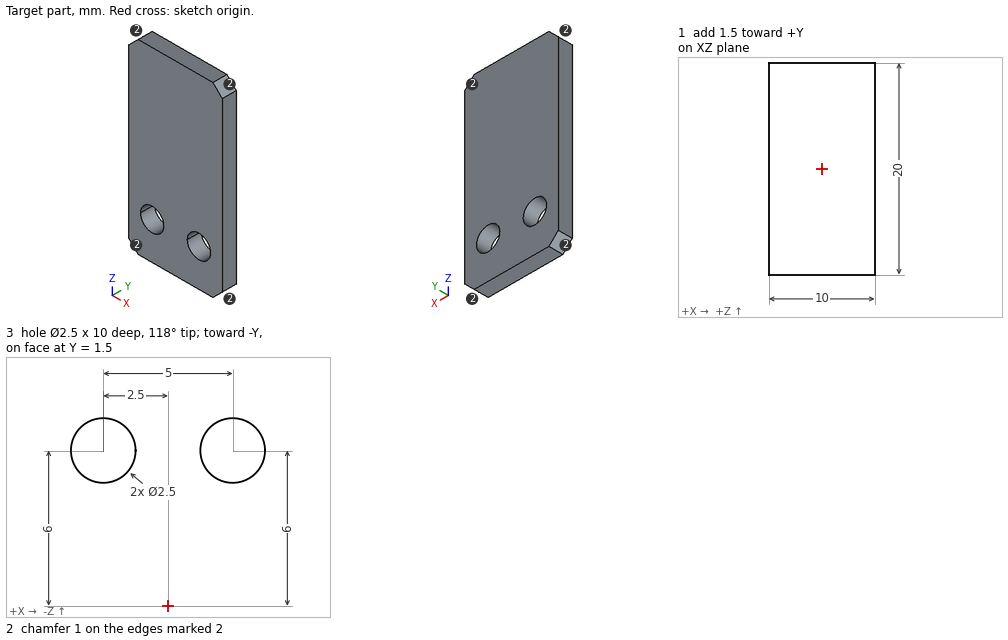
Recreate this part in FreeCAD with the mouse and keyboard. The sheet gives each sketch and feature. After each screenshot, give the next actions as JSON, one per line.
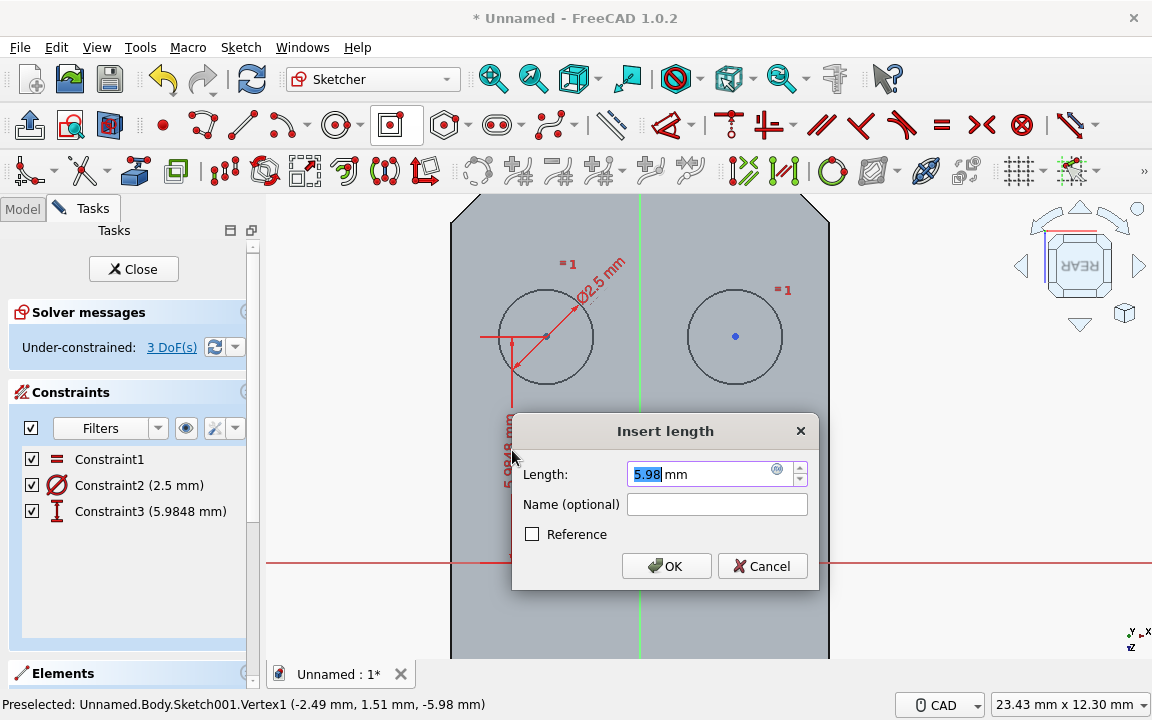
{"action": "type", "text": "6"}
{"action": "key", "text": "Return"}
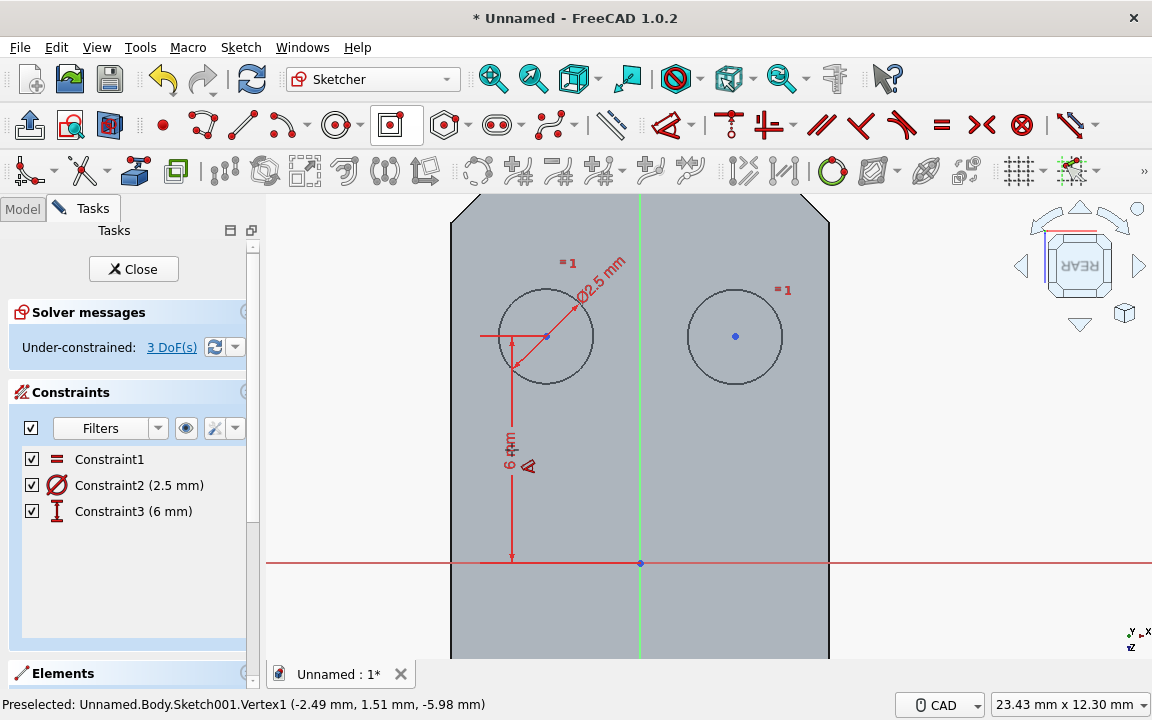
{"action": "left_click", "coordinate": [735, 337]}
{"action": "left_click", "coordinate": [769, 450]}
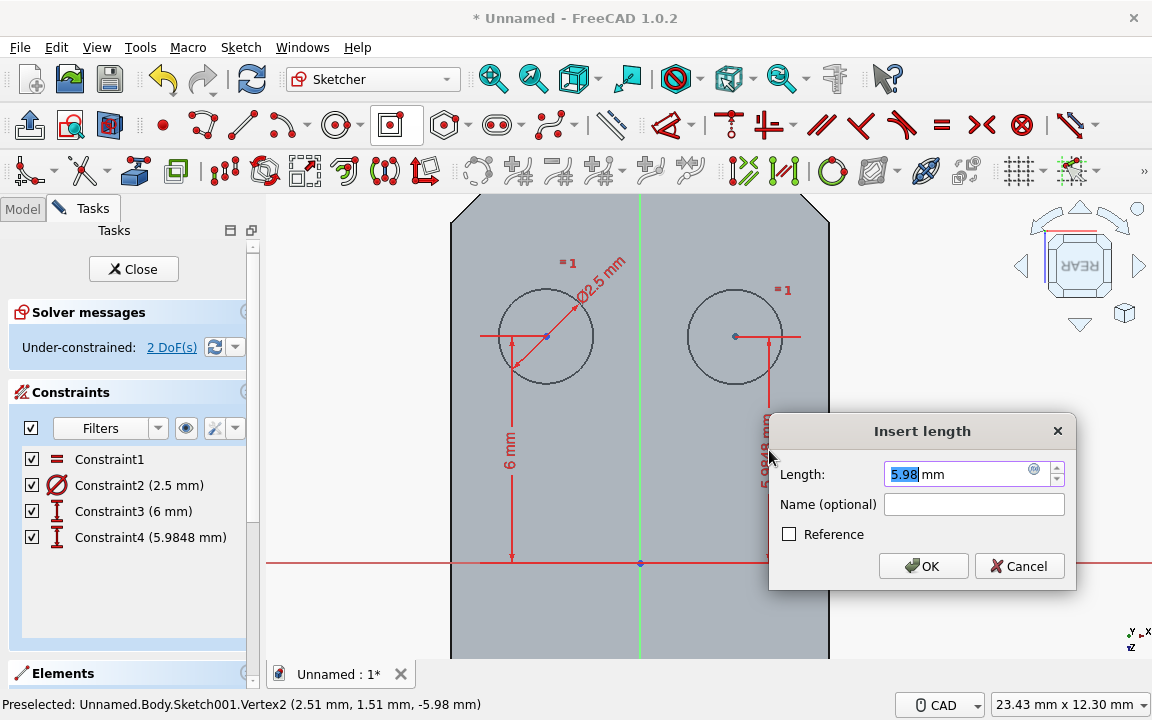
{"action": "type", "text": "6"}
{"action": "key", "text": "Return"}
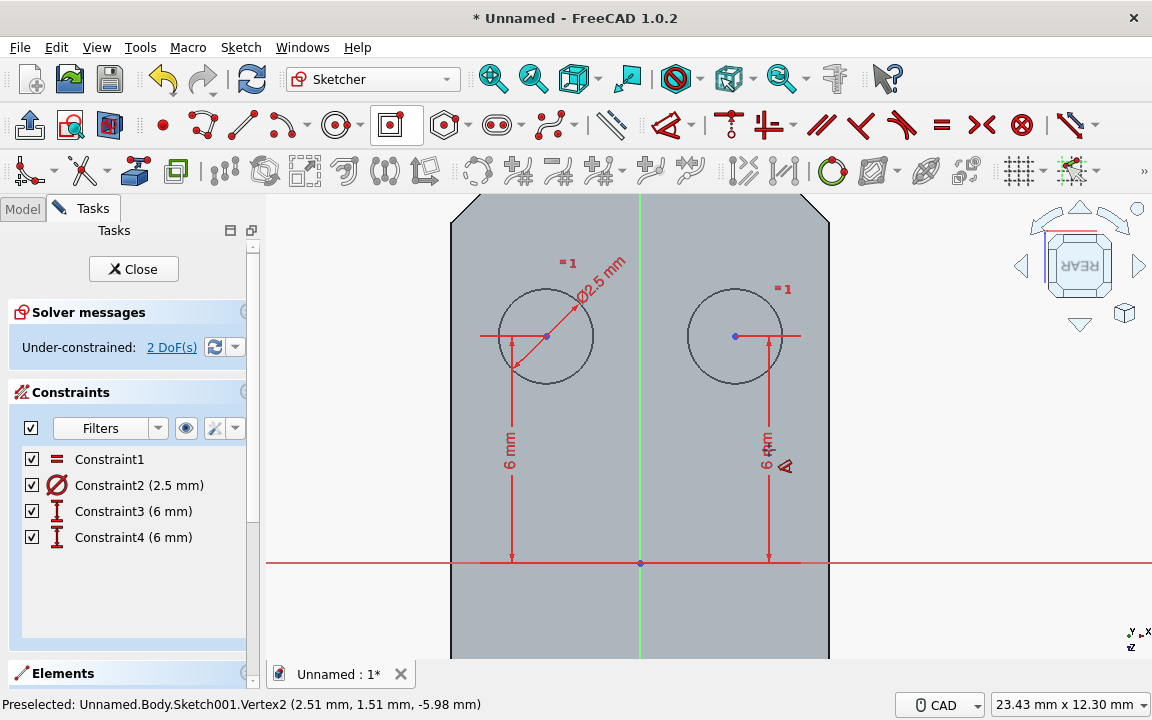
{"action": "left_click", "coordinate": [546, 336]}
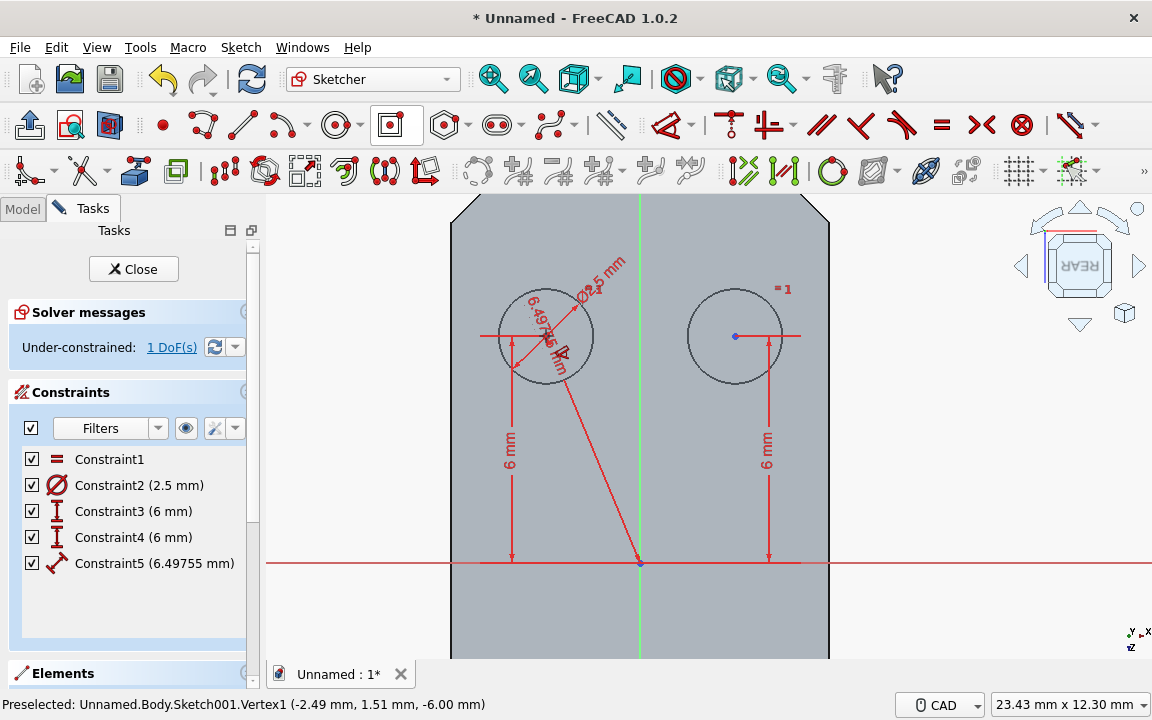
{"action": "left_click", "coordinate": [735, 336]}
{"action": "left_click", "coordinate": [597, 302]}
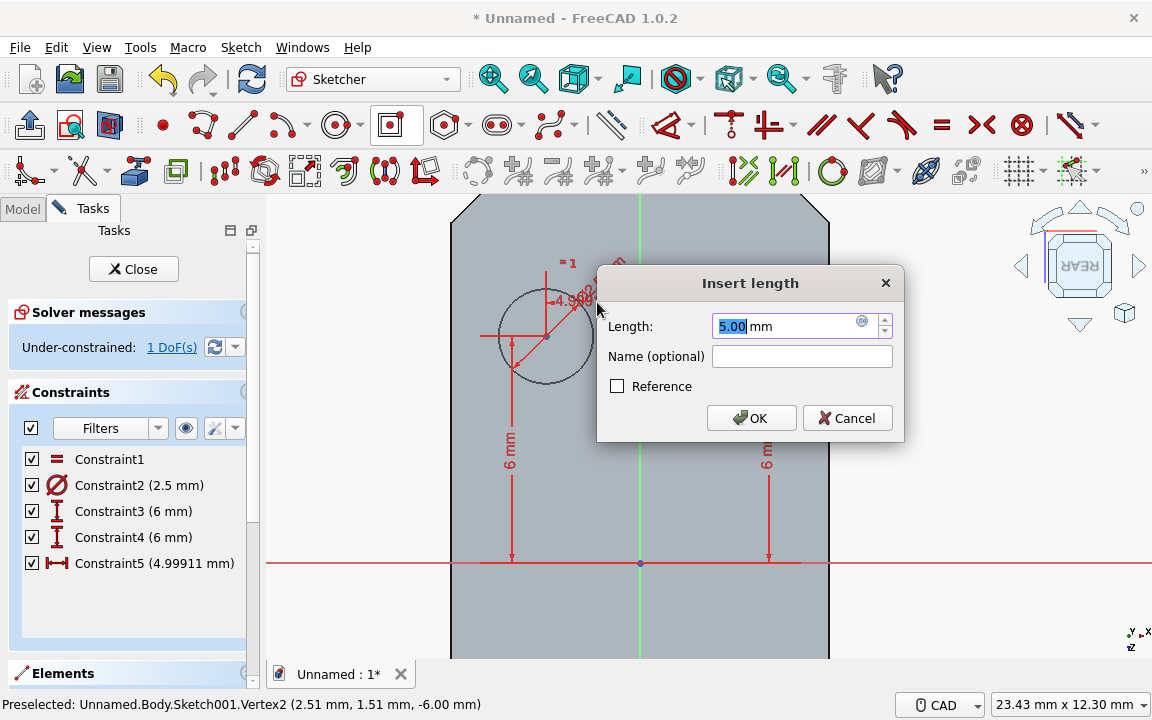
{"action": "type", "text": "5"}
{"action": "key", "text": "Return"}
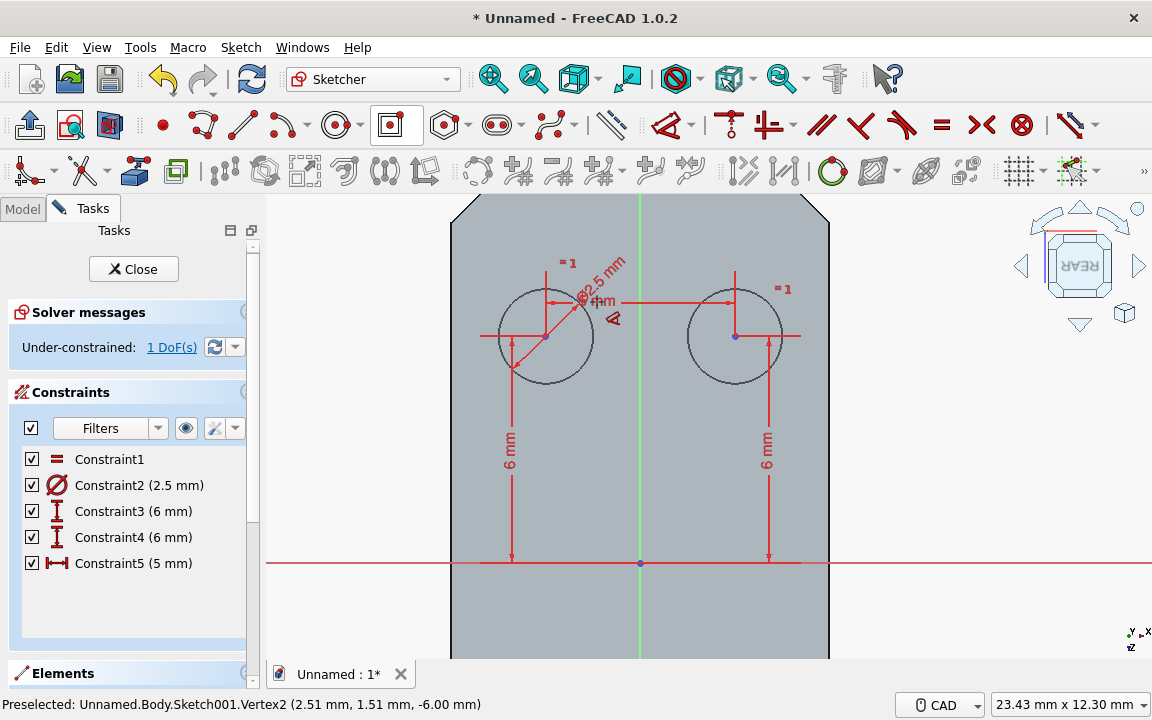
{"action": "left_click", "coordinate": [546, 336]}
{"action": "left_click", "coordinate": [593, 597]}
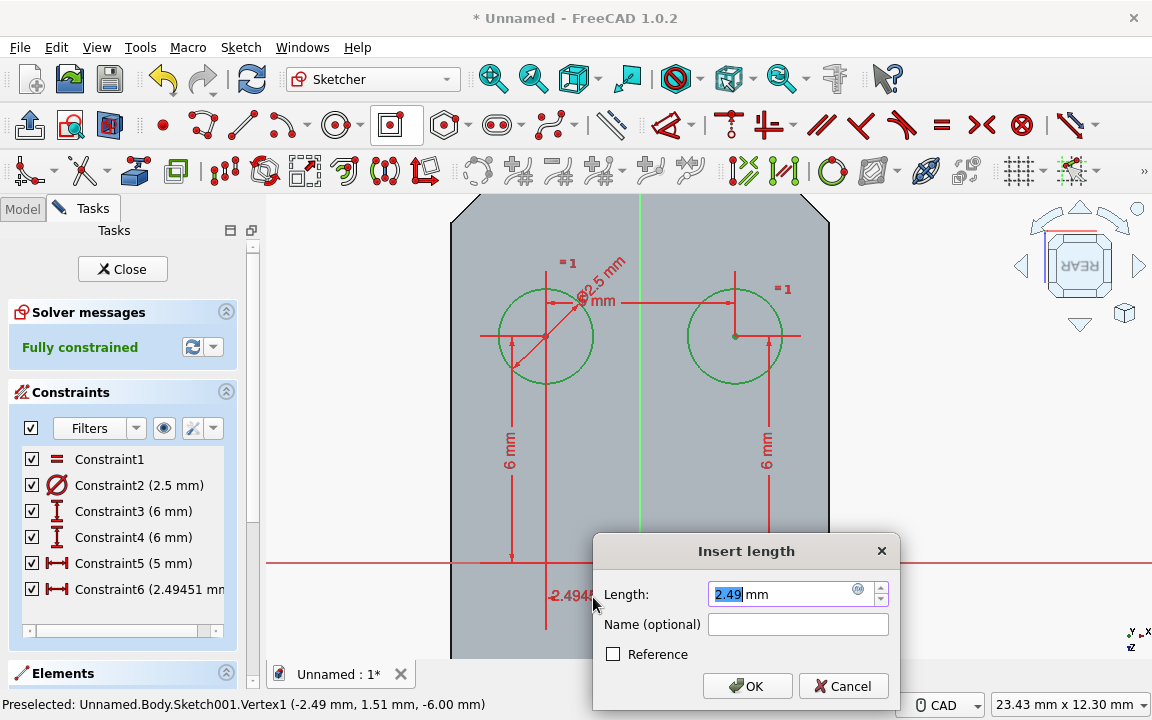
{"action": "type", "text": "2.5"}
{"action": "key", "text": "Return"}
{"action": "key", "text": "Escape"}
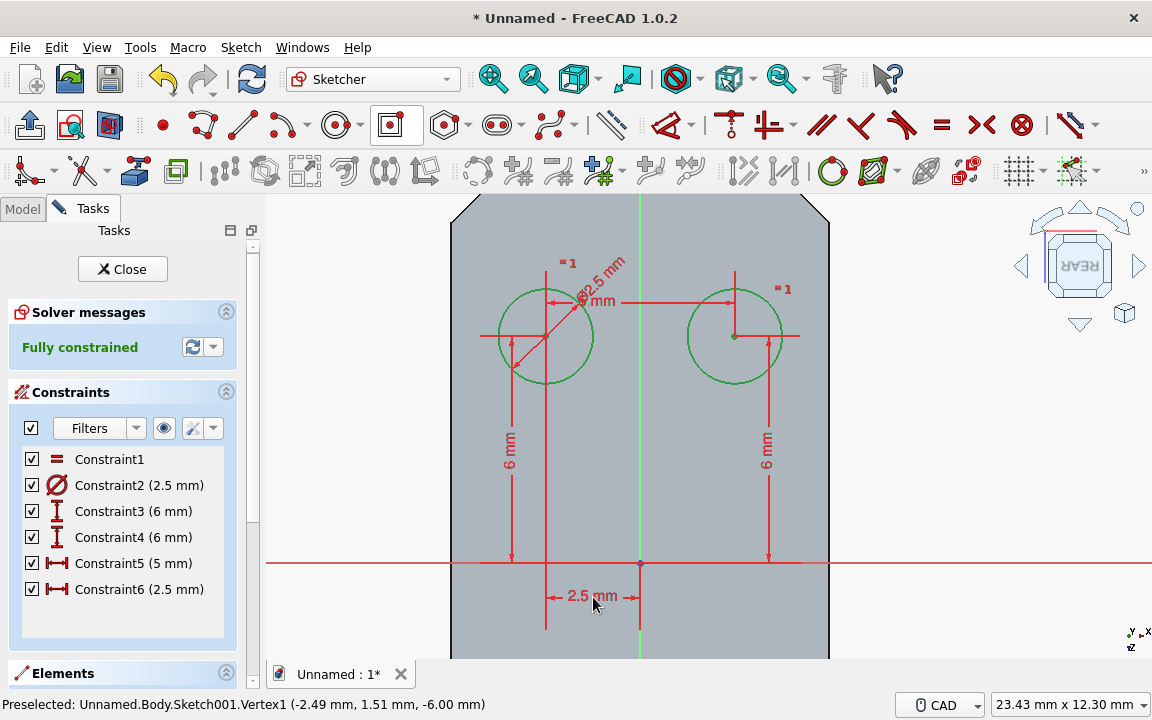
{"action": "left_click", "coordinate": [123, 269]}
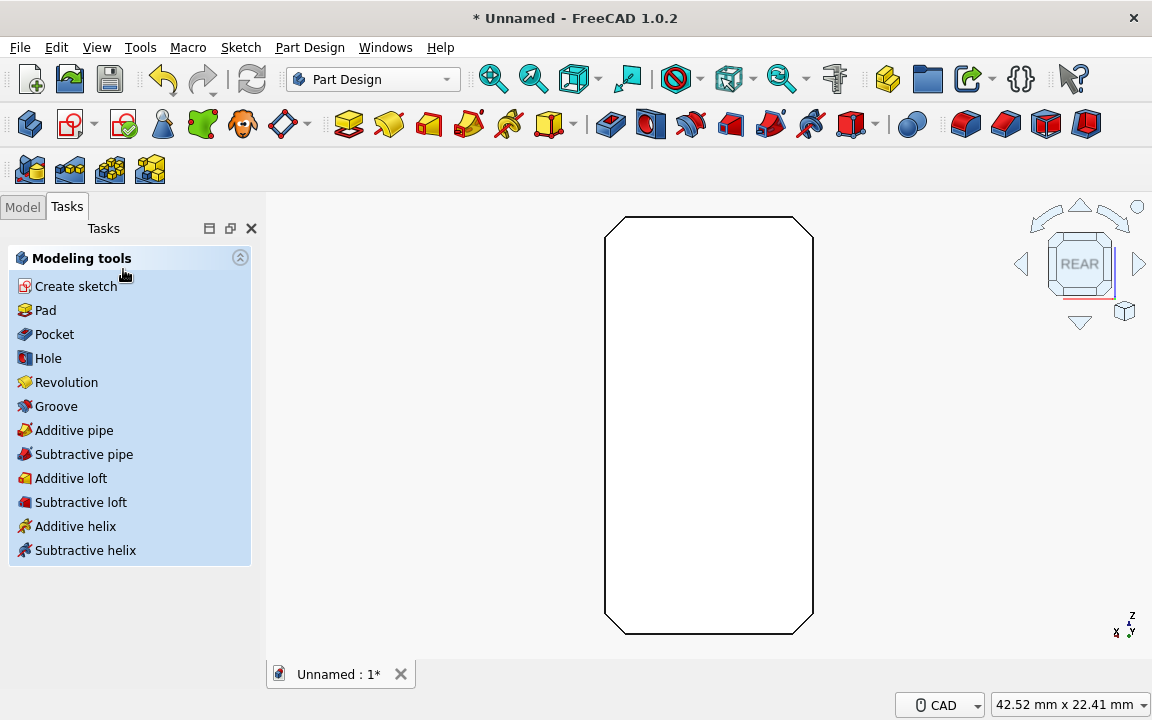
{"action": "left_click", "coordinate": [652, 124]}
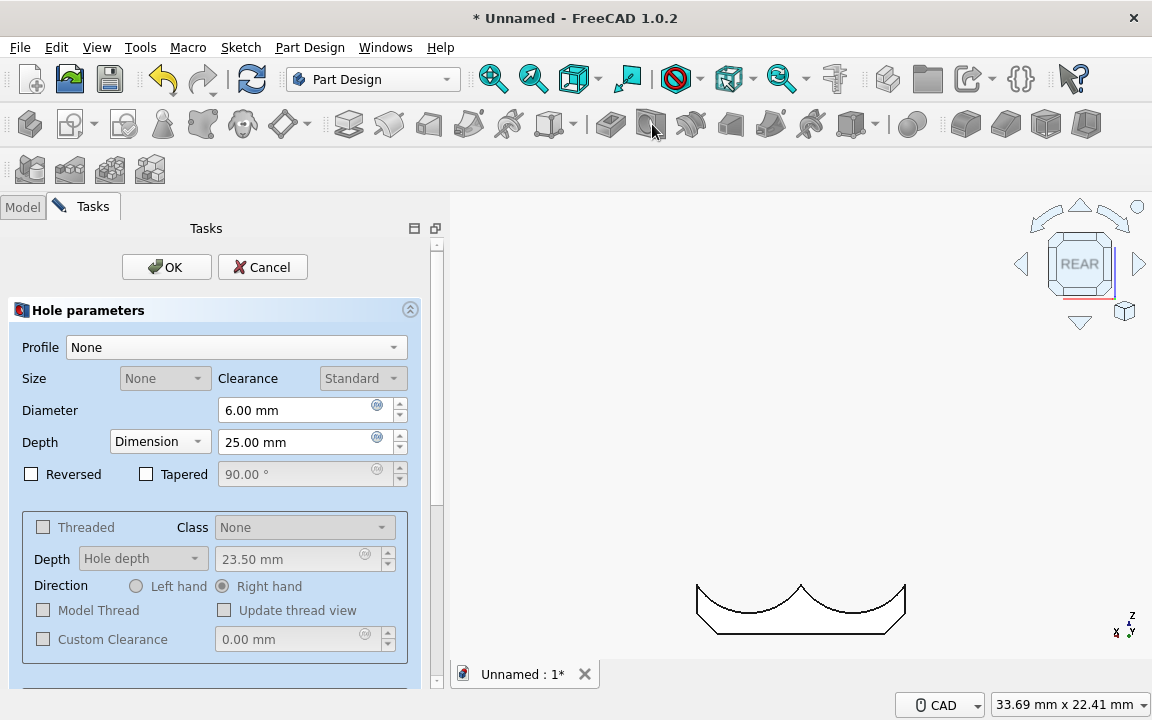
{"action": "triple_click", "coordinate": [305, 410]}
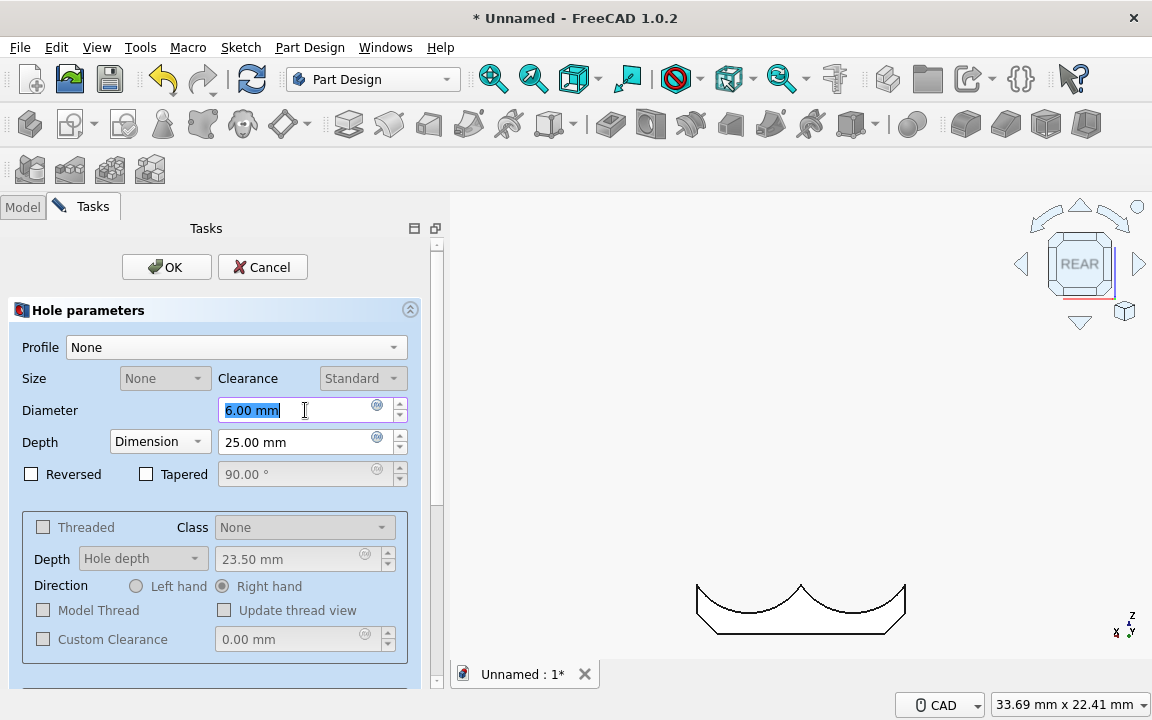
{"action": "type", "text": "2.5"}
{"action": "key", "text": "Tab"}